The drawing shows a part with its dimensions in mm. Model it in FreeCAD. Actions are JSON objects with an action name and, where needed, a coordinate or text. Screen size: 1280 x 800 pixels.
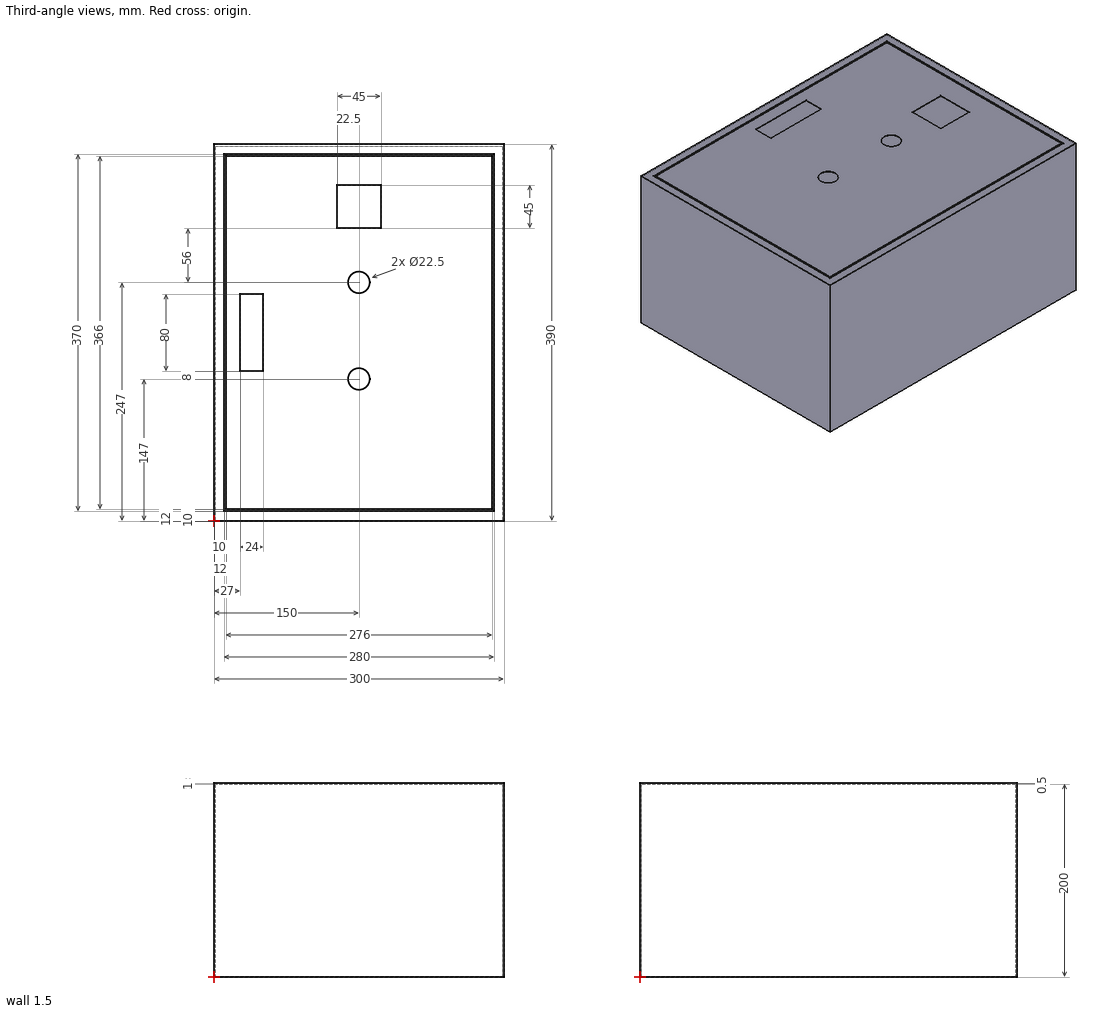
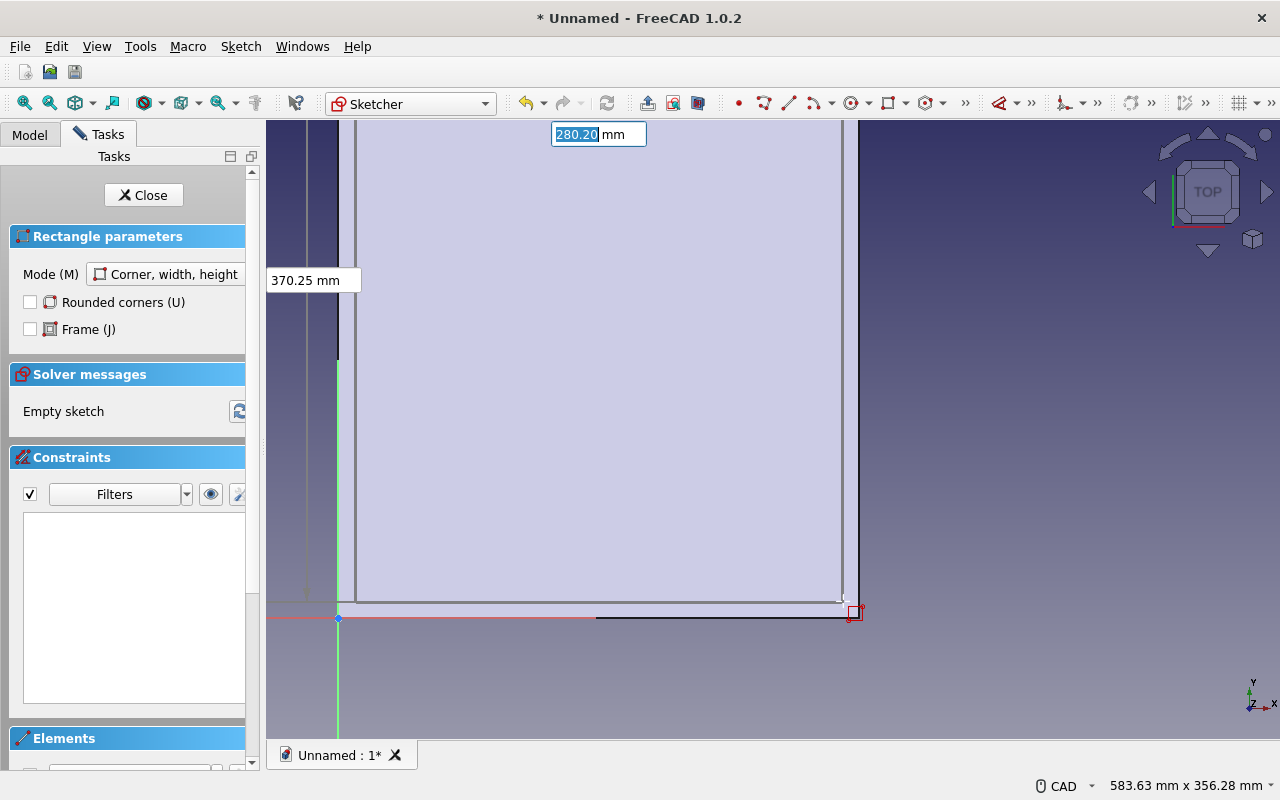
{"action": "left_click", "coordinate": [842, 601]}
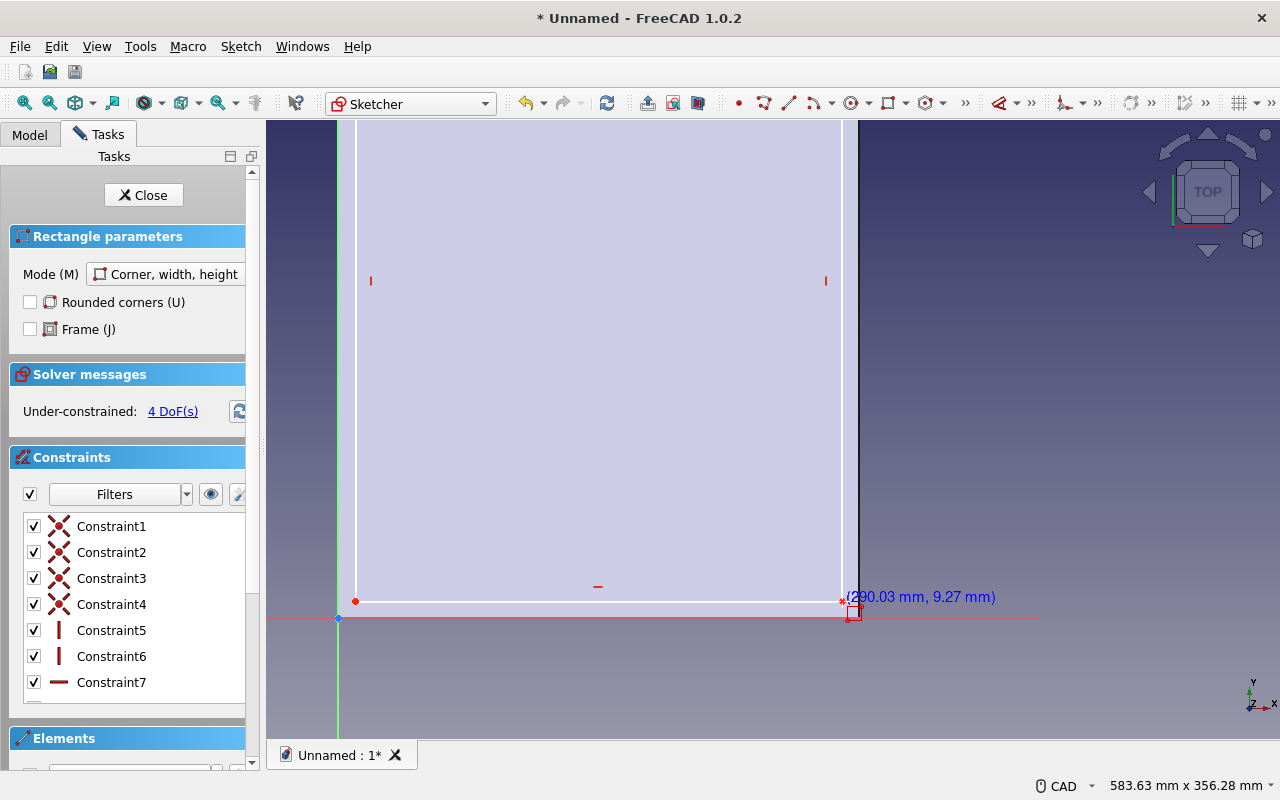
{"action": "left_click", "coordinate": [385, 210]}
{"action": "mouse_move", "coordinate": [427, 349]}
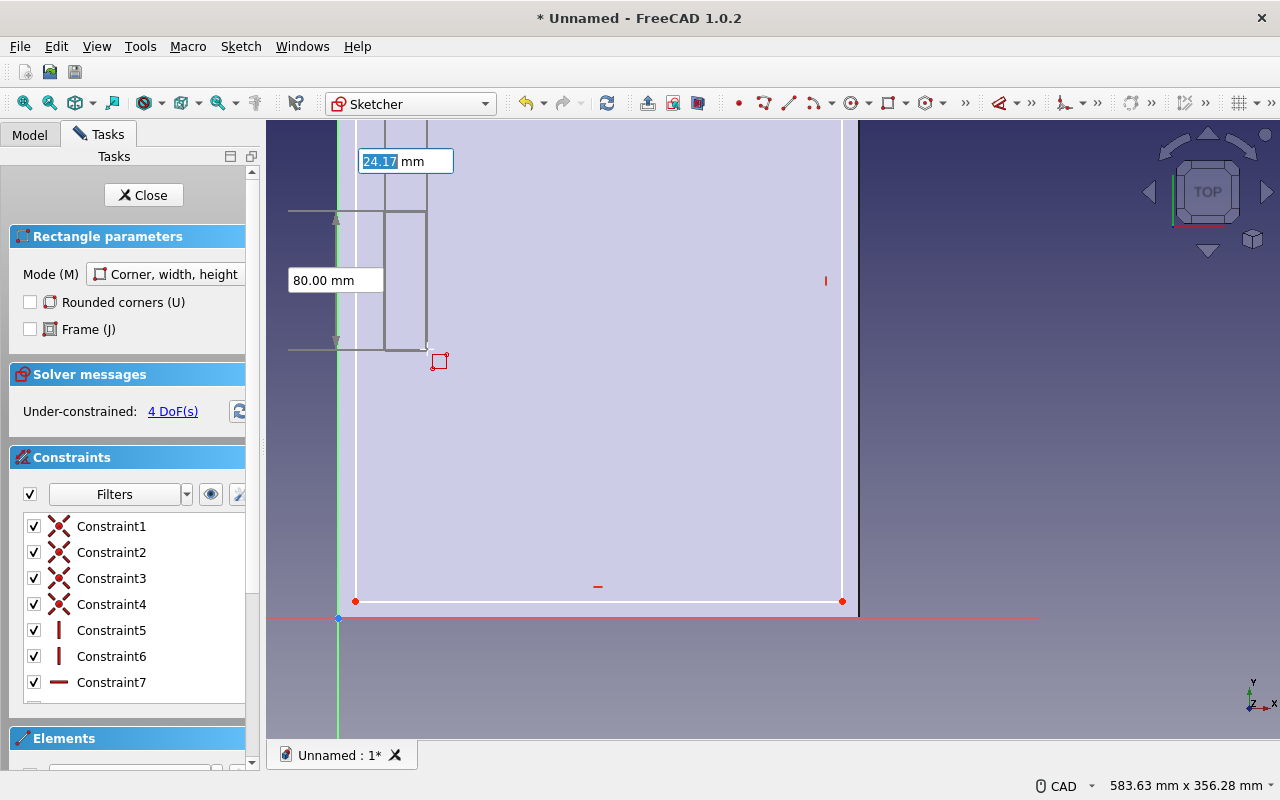
{"action": "type", "text": "24"}
{"action": "key", "text": "Tab"}
{"action": "type", "text": "80"}
{"action": "key", "text": "Return"}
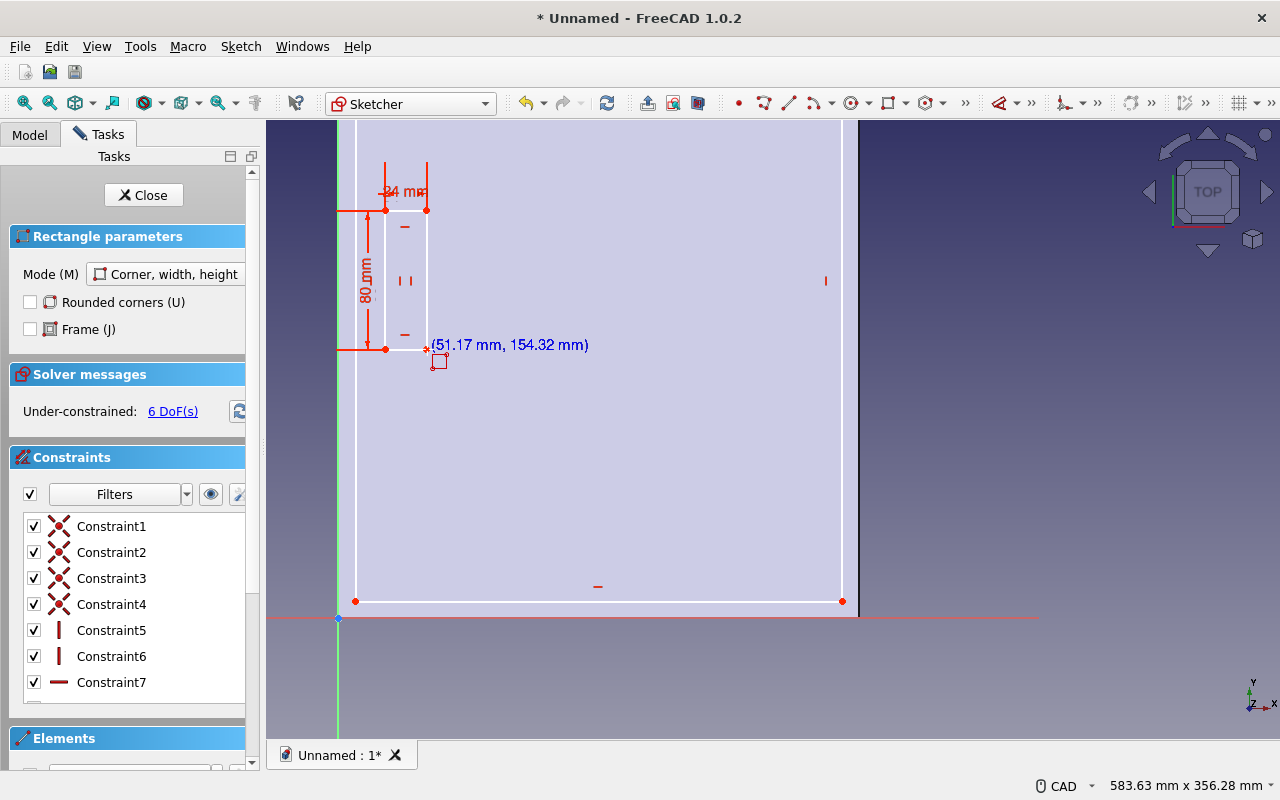
{"action": "scroll", "coordinate": [844, 602], "scroll_direction": "down", "scroll_amount": 3}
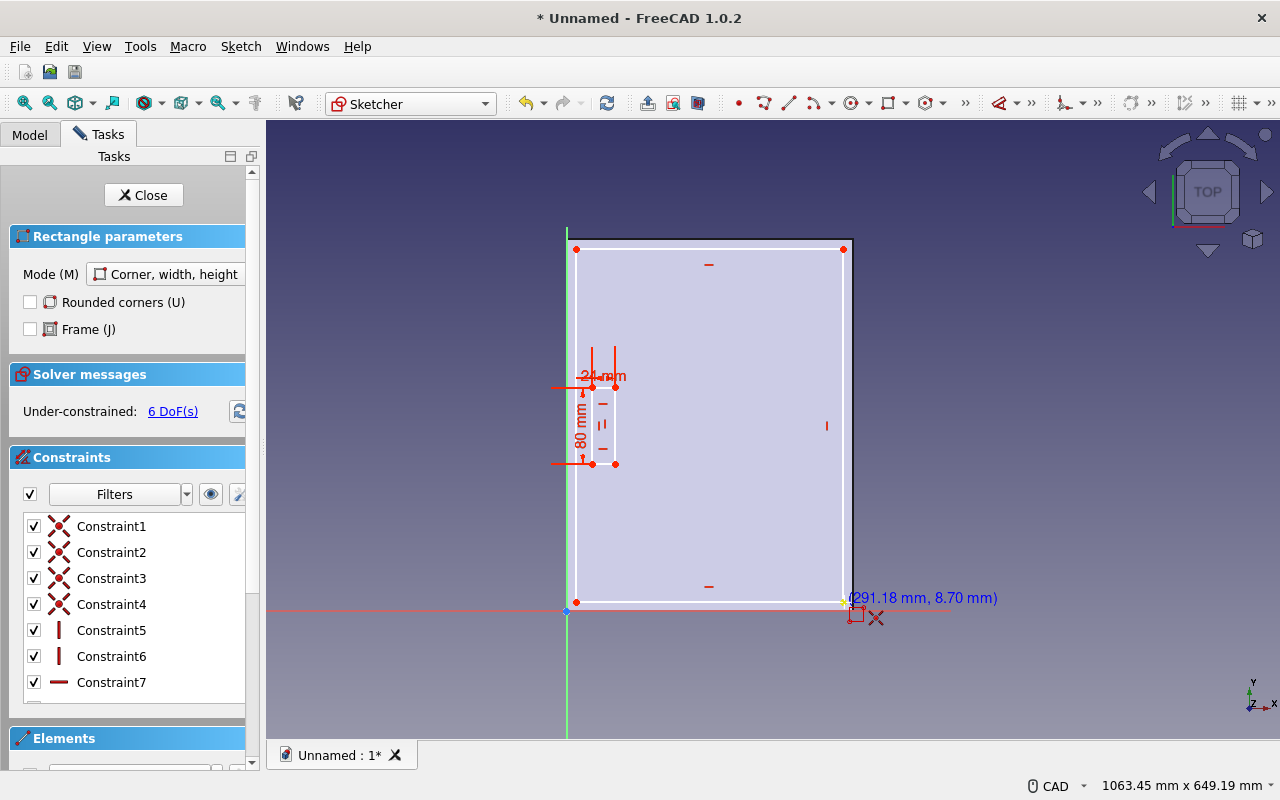
{"action": "left_click", "coordinate": [688, 279]}
{"action": "mouse_move", "coordinate": [731, 322]}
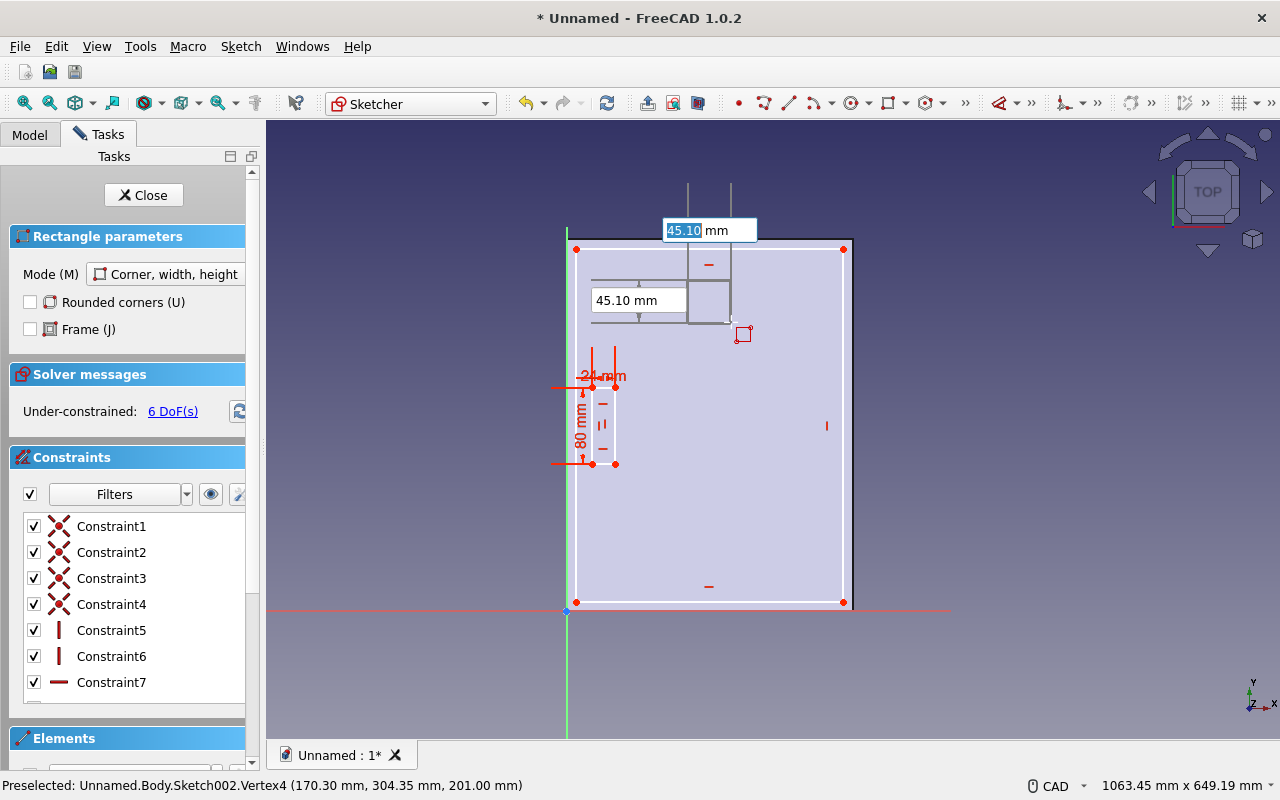
{"action": "type", "text": "45"}
{"action": "key", "text": "Tab"}
{"action": "type", "text": "45"}
{"action": "key", "text": "Return"}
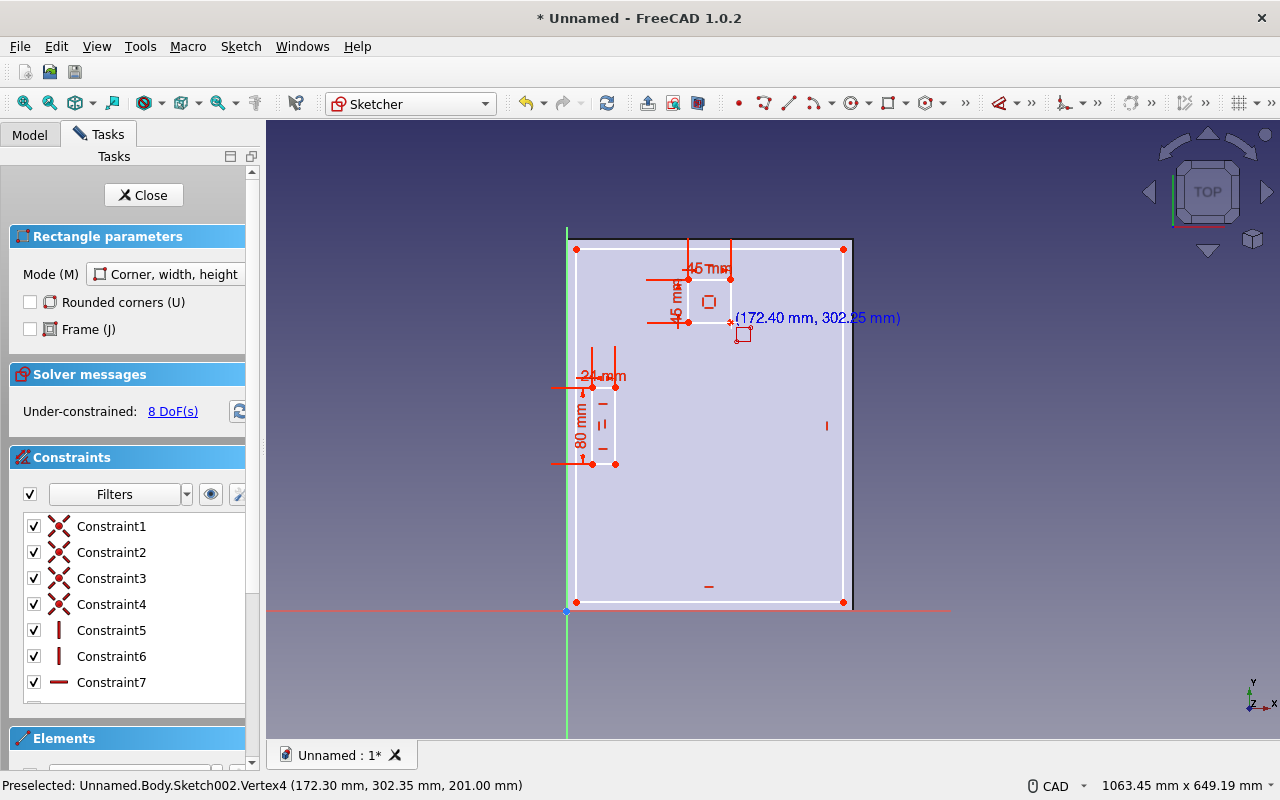
{"action": "scroll", "coordinate": [578, 251], "scroll_direction": "up", "scroll_amount": 11}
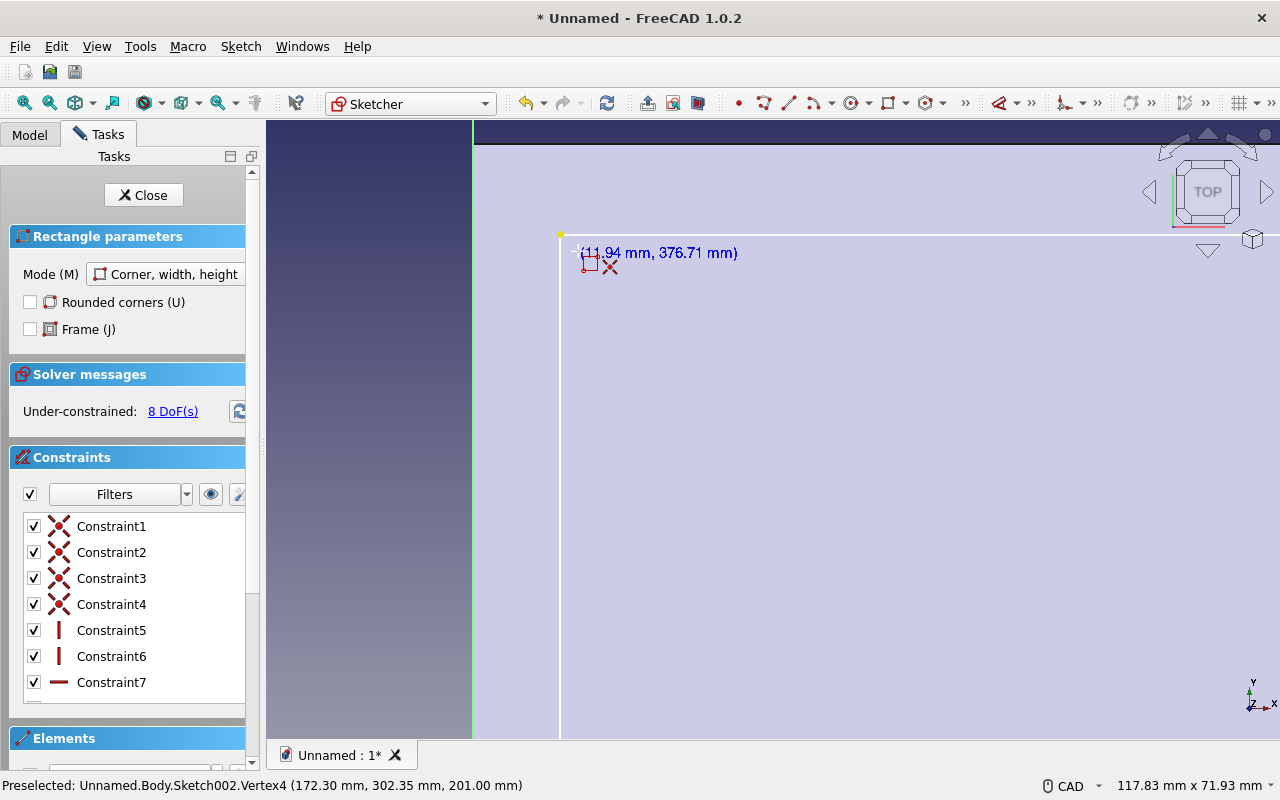
{"action": "left_click", "coordinate": [576, 247]}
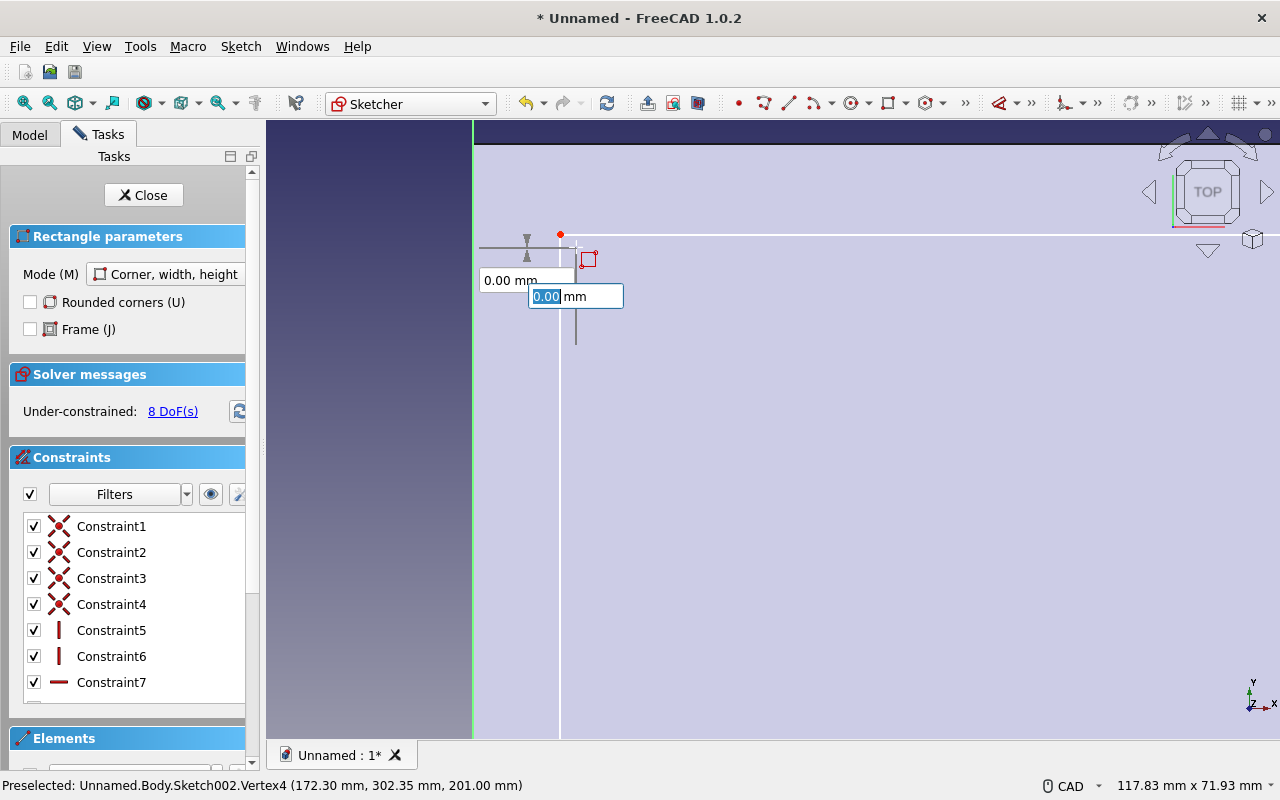
{"action": "scroll", "coordinate": [578, 251], "scroll_direction": "down", "scroll_amount": 11}